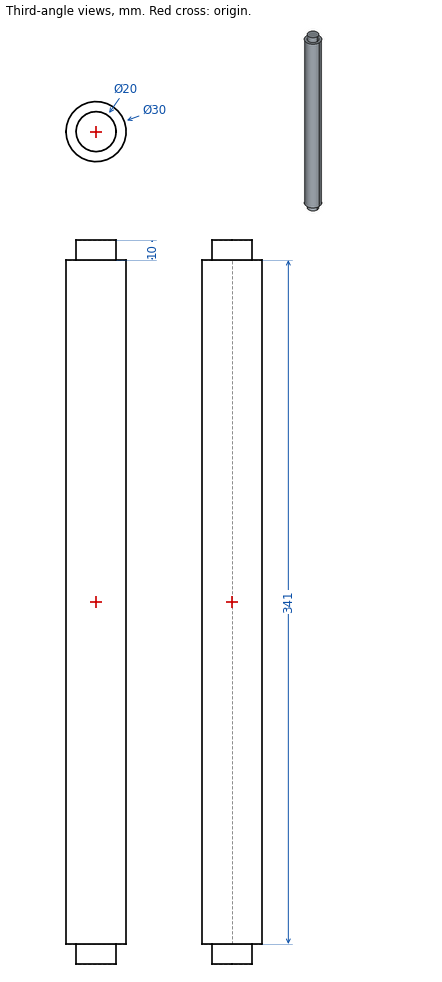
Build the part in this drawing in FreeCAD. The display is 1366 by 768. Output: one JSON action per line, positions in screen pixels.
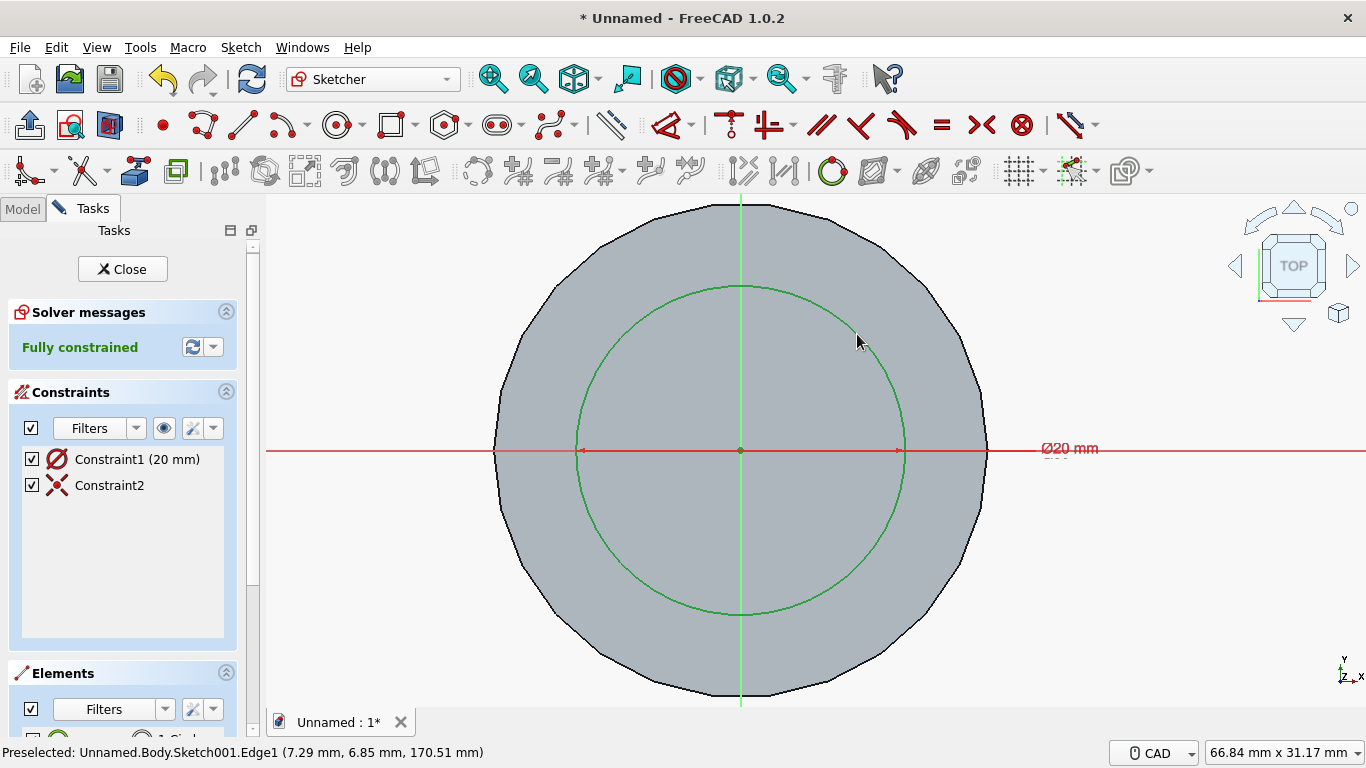
{"action": "left_click", "coordinate": [123, 269]}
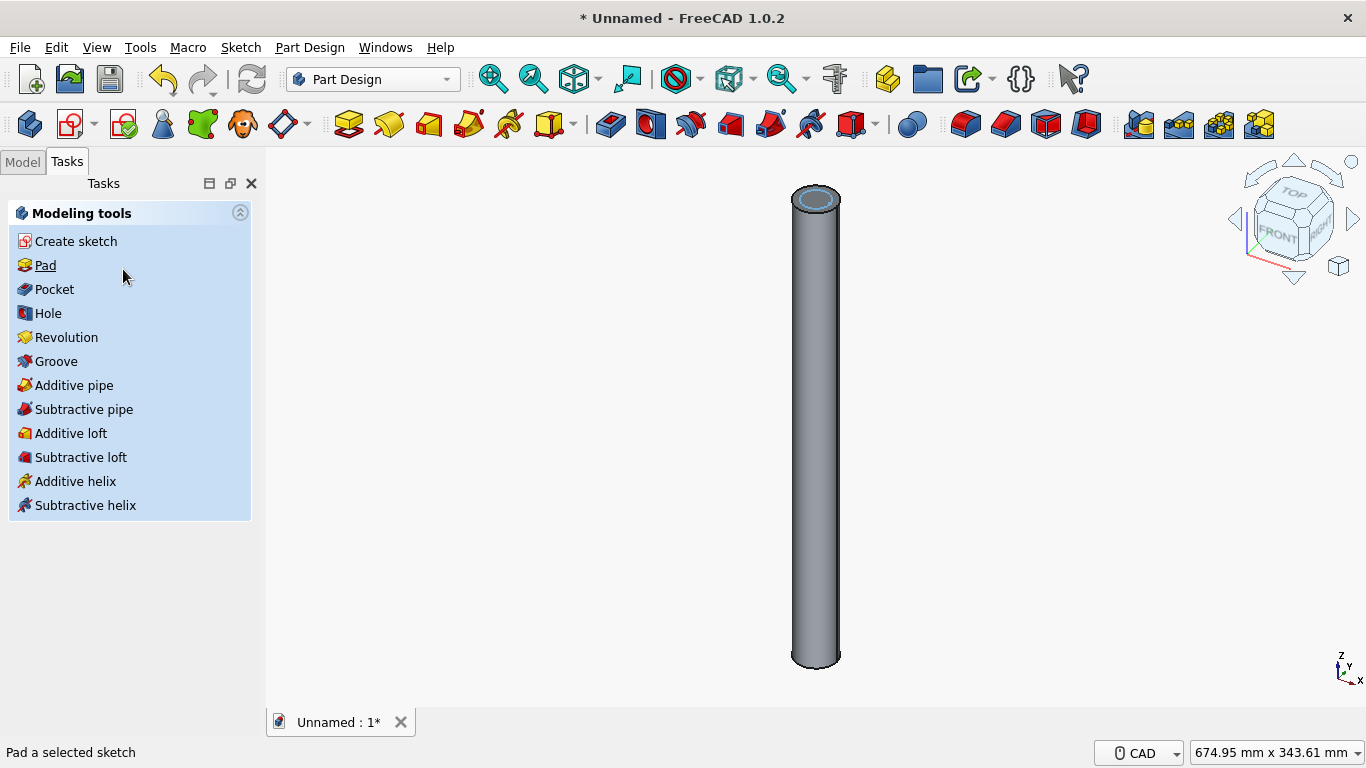
{"action": "left_click", "coordinate": [350, 124]}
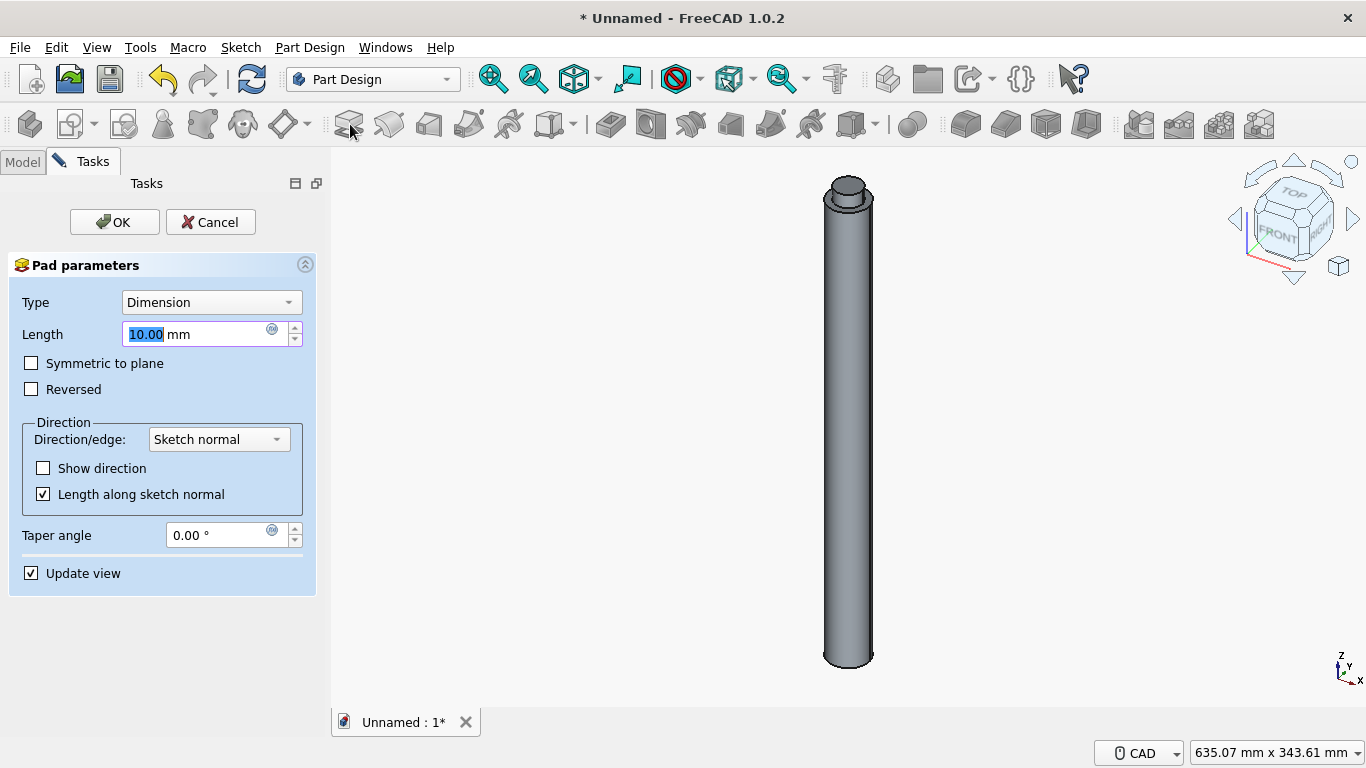
{"action": "type", "text": "10"}
{"action": "key", "text": "Tab"}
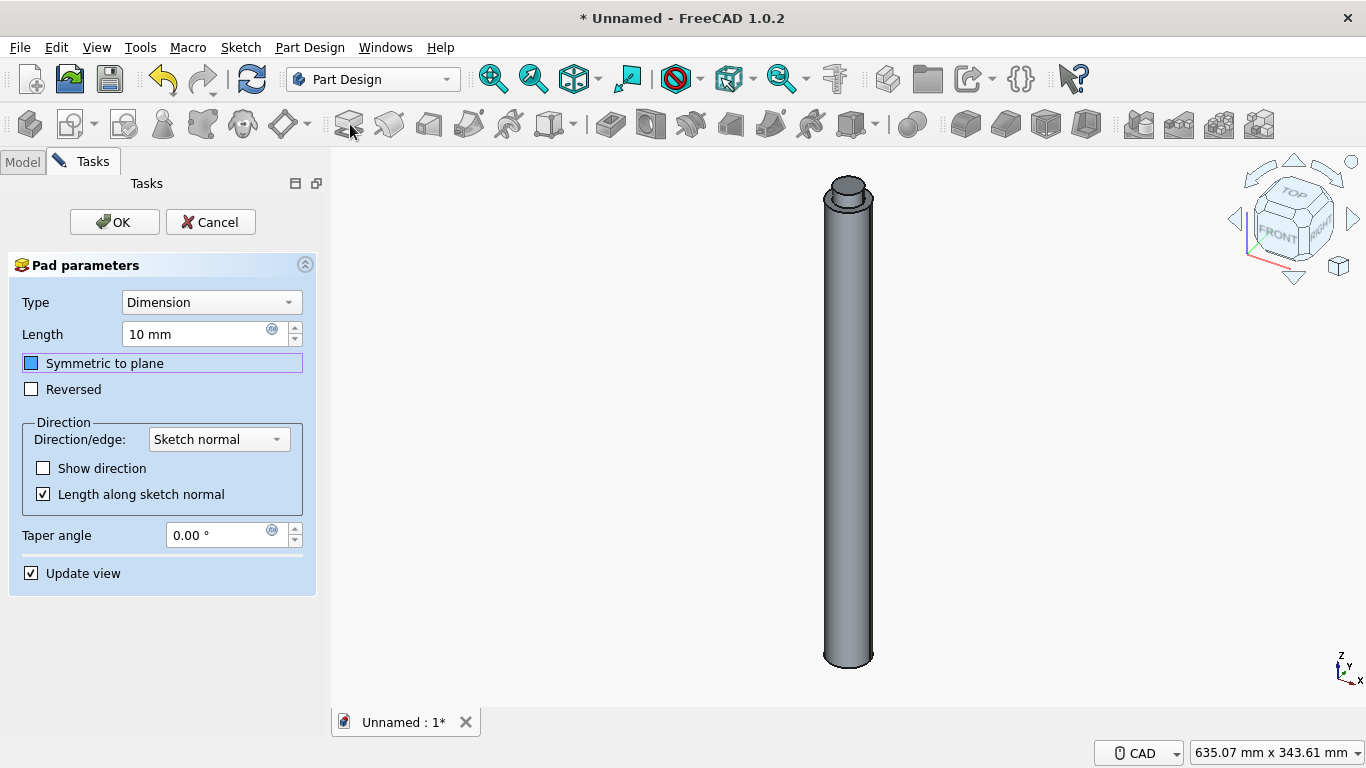
{"action": "left_click", "coordinate": [115, 222]}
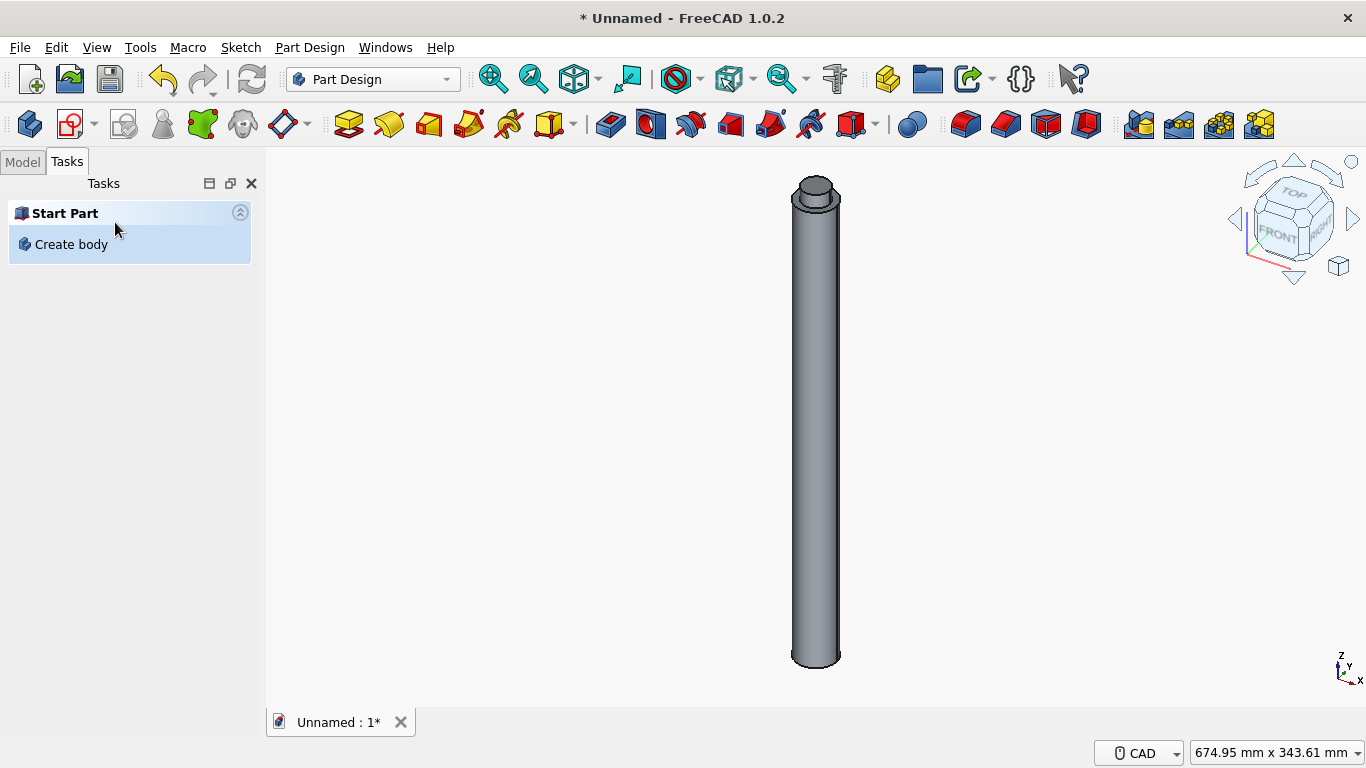
{"action": "left_click", "coordinate": [23, 161]}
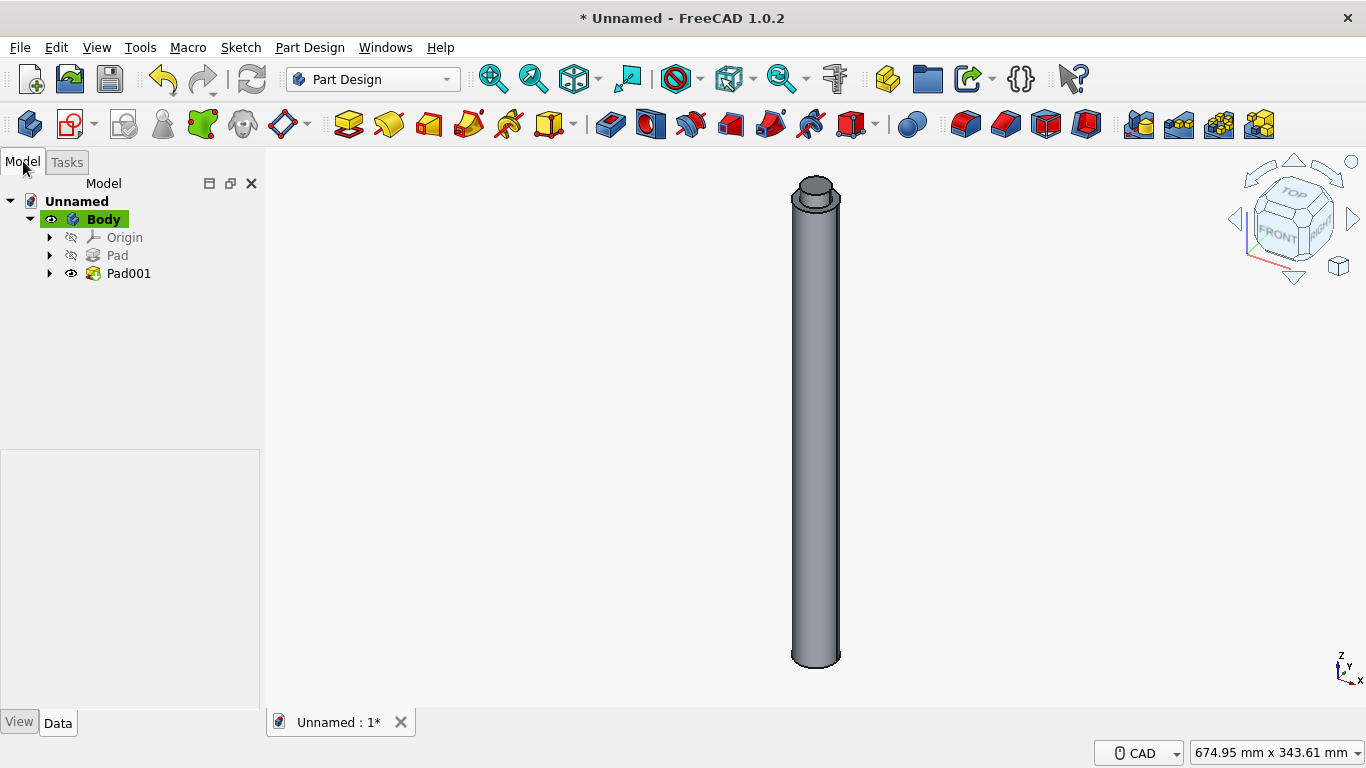
{"action": "left_click", "coordinate": [116, 273]}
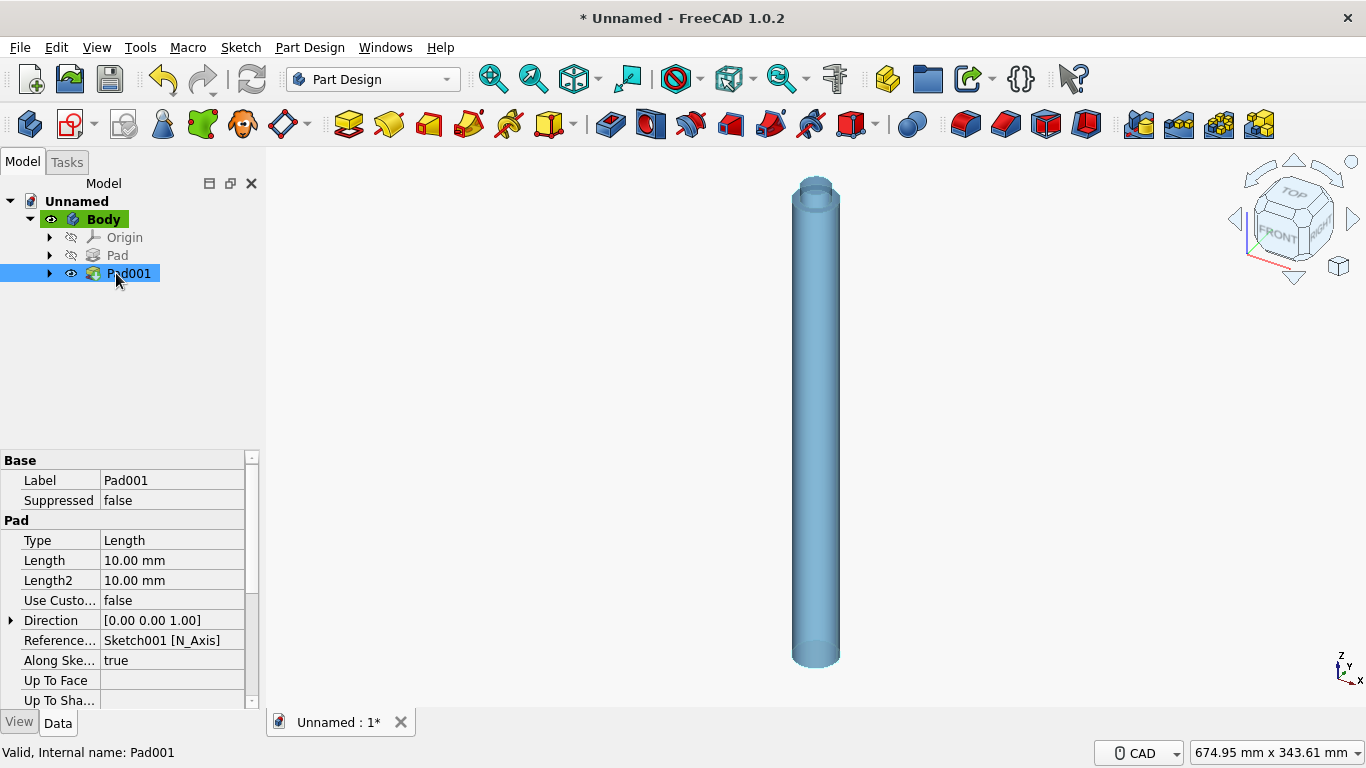
{"action": "left_click", "coordinate": [1140, 124]}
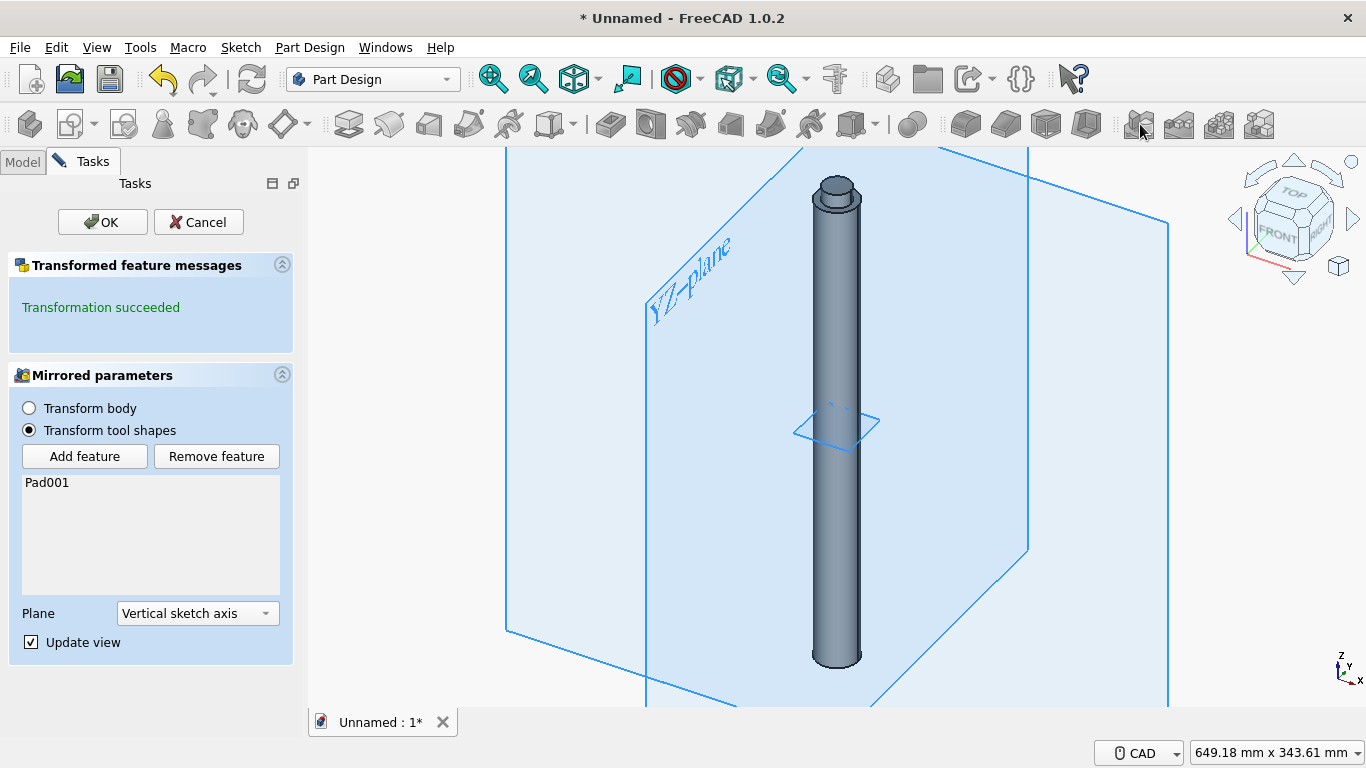
{"action": "left_click", "coordinate": [198, 614]}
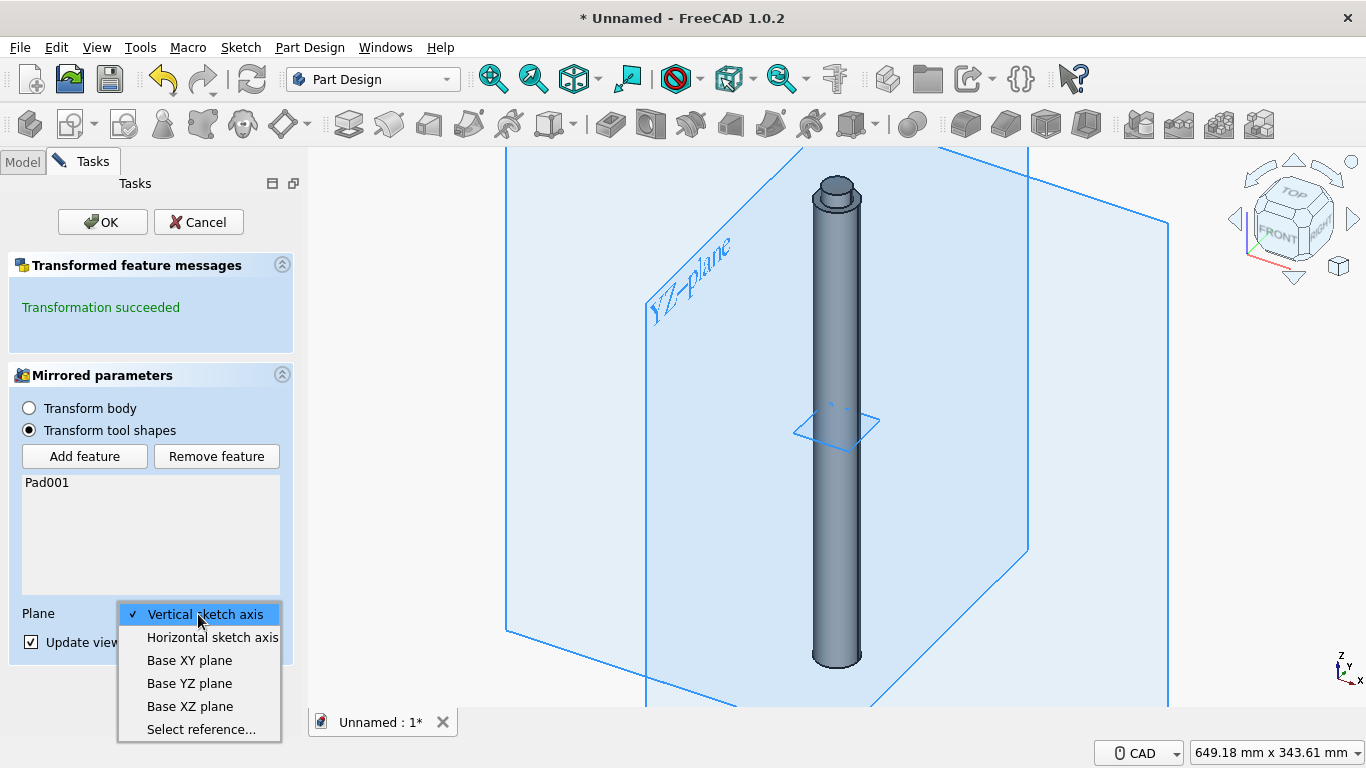
{"action": "left_click", "coordinate": [198, 660]}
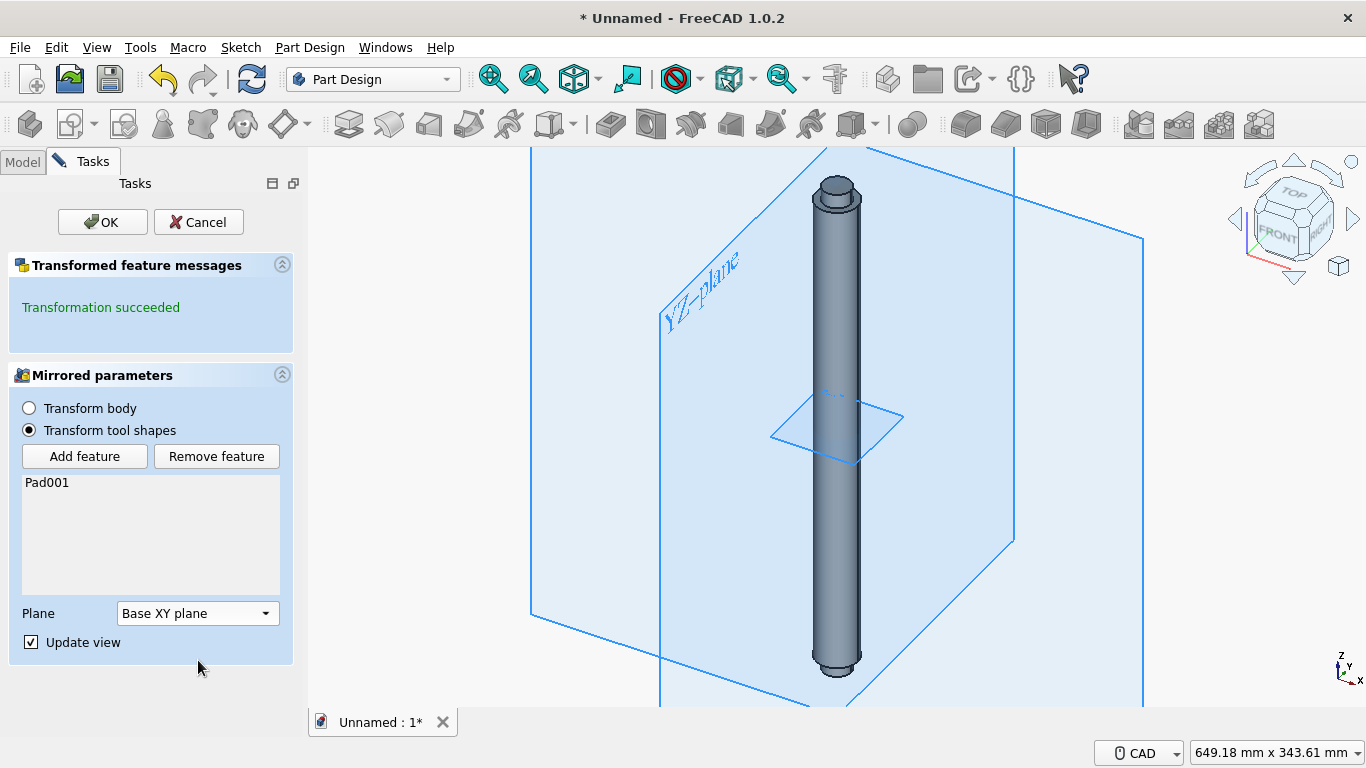
{"action": "left_click", "coordinate": [103, 222]}